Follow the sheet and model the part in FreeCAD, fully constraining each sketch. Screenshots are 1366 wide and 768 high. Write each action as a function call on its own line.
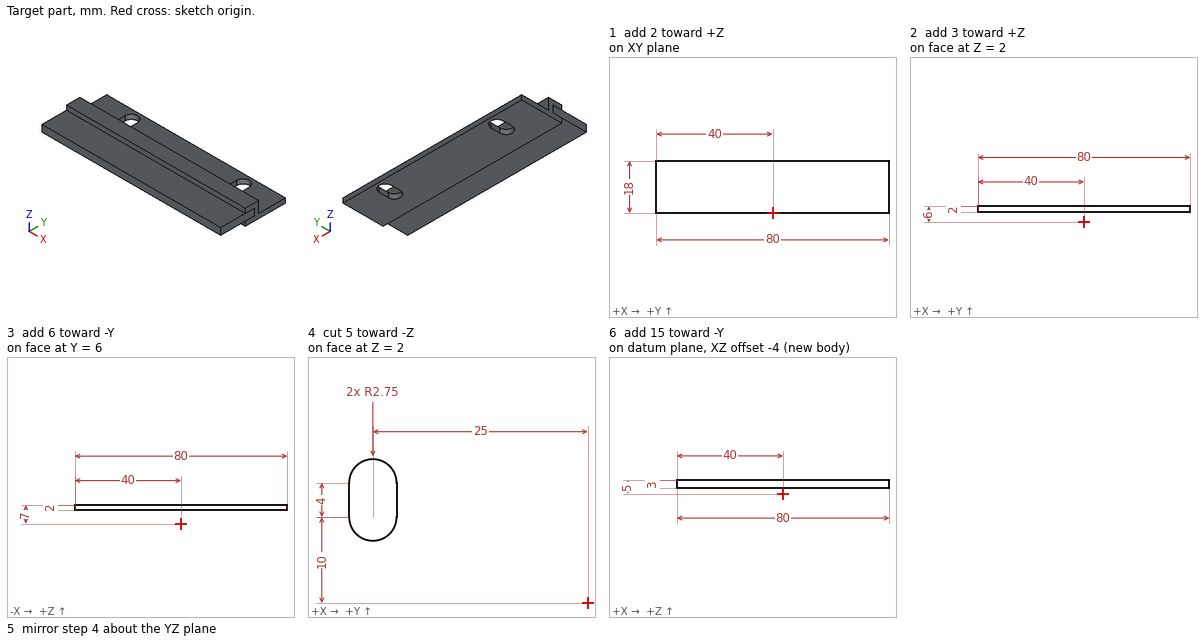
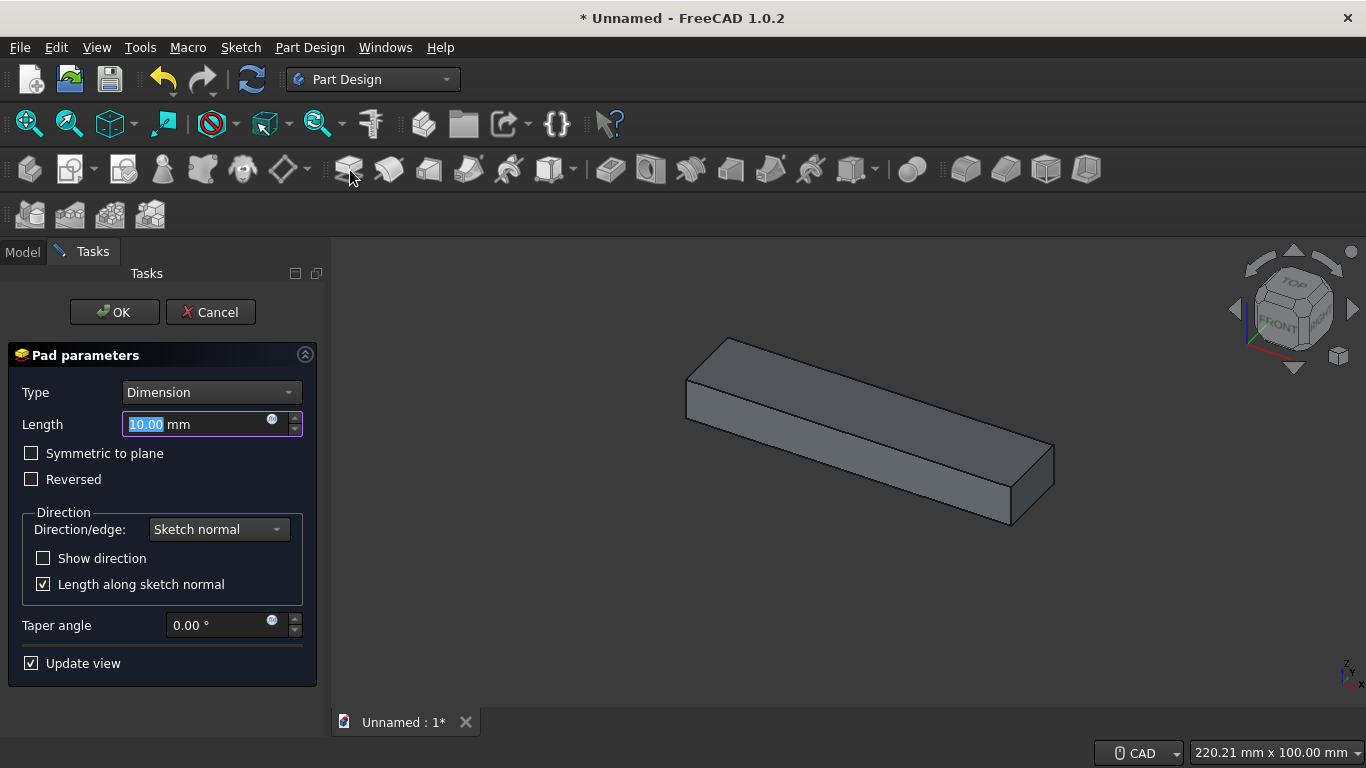
text(2)
key(Tab)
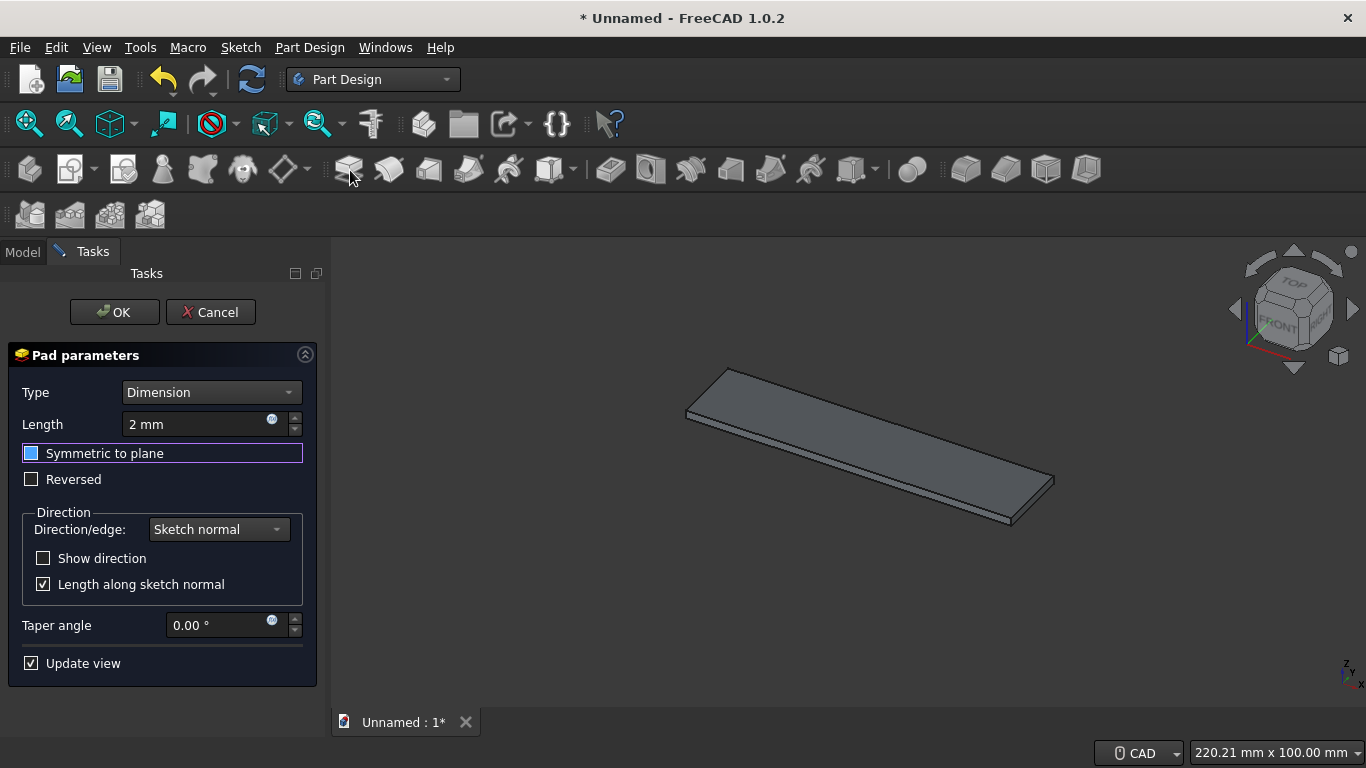
click(115, 312)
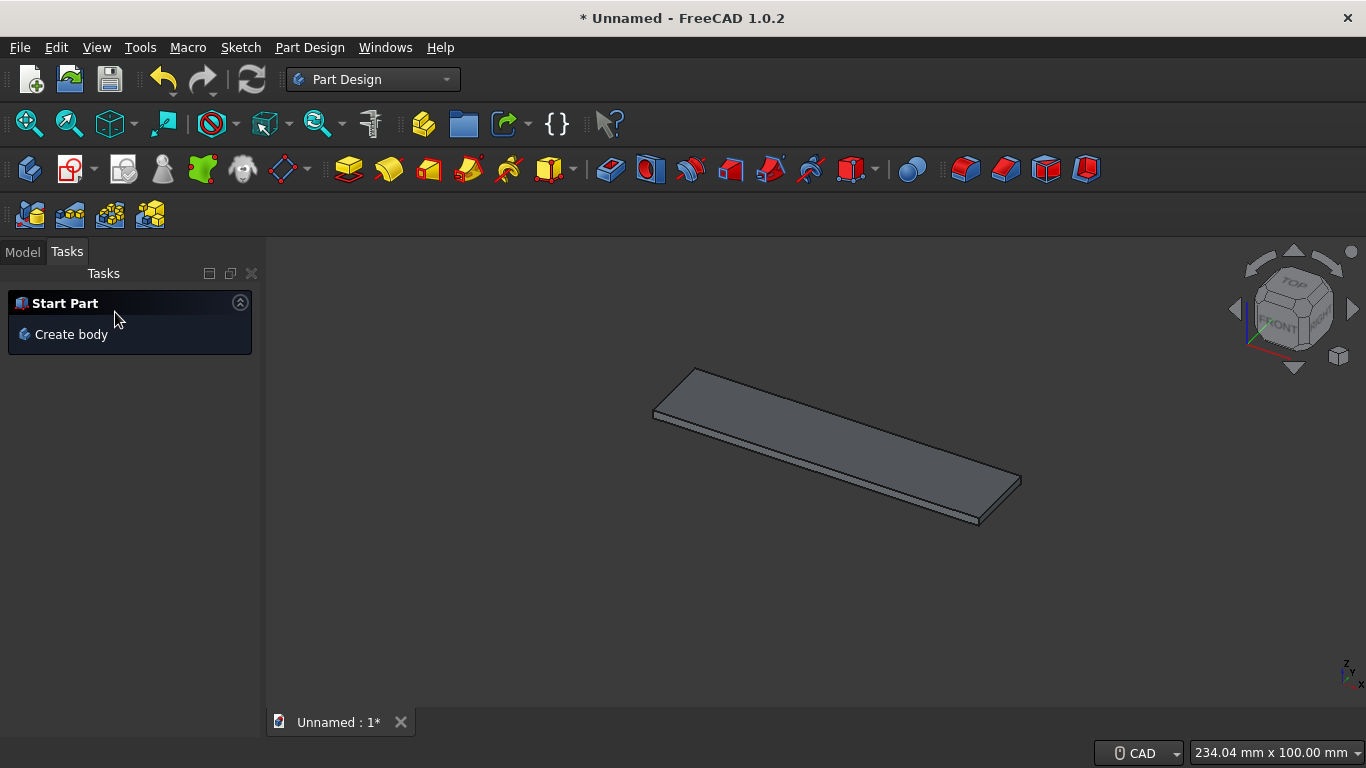
click(30, 124)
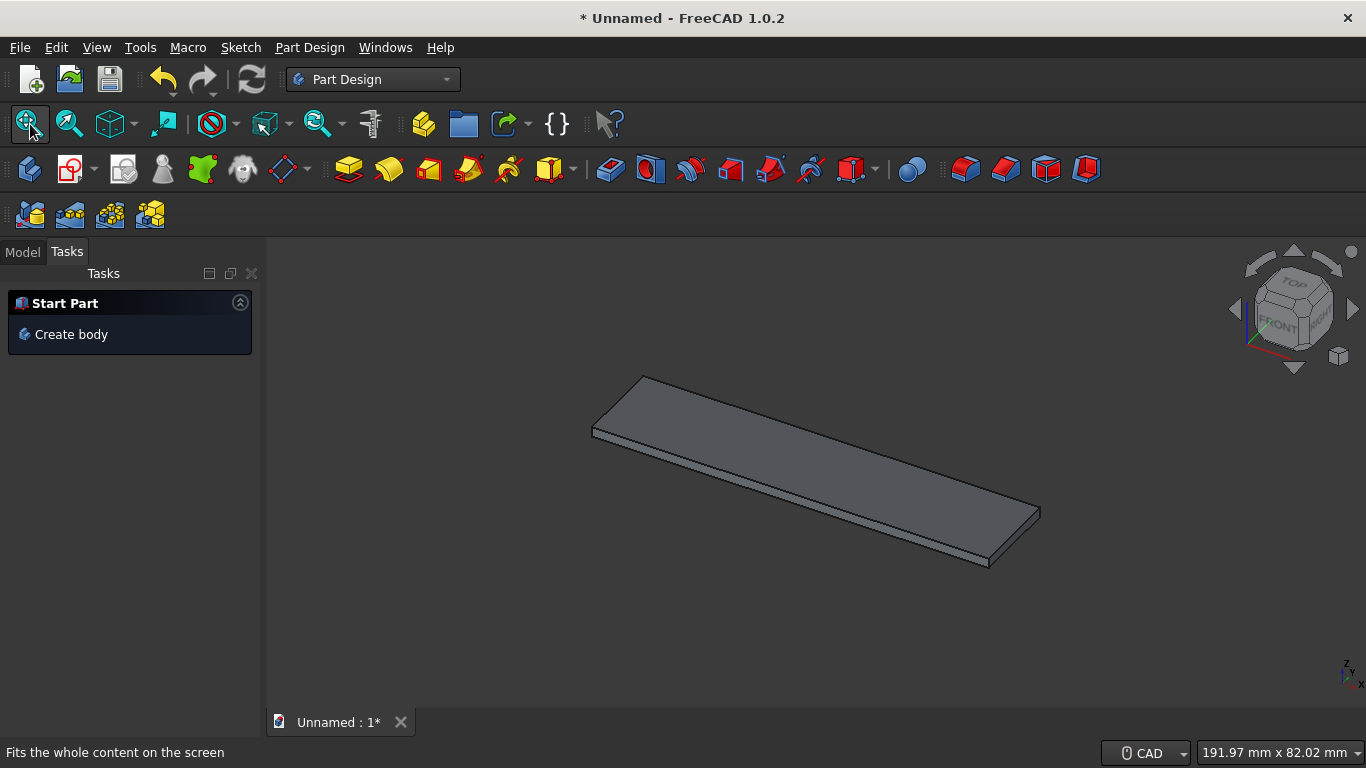
click(929, 504)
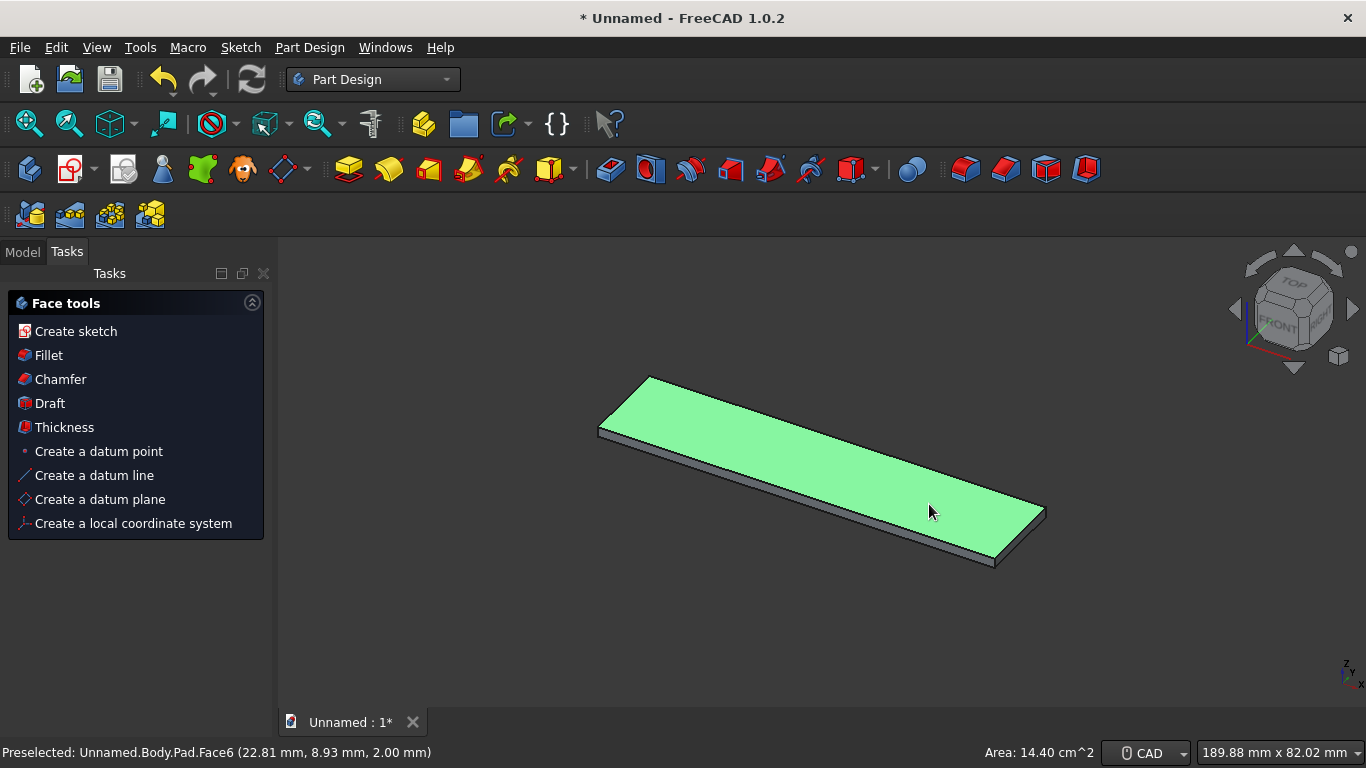
click(70, 170)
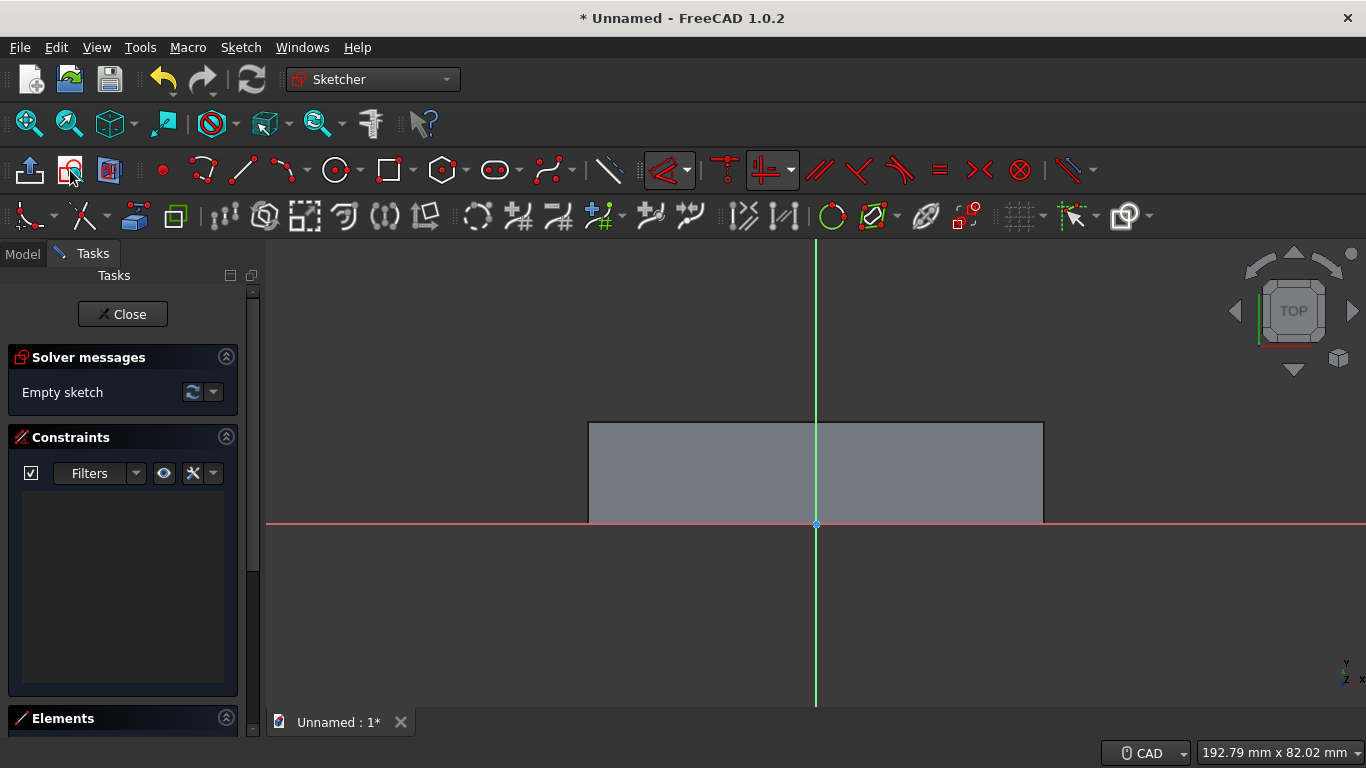
scroll(955, 577, up, 2)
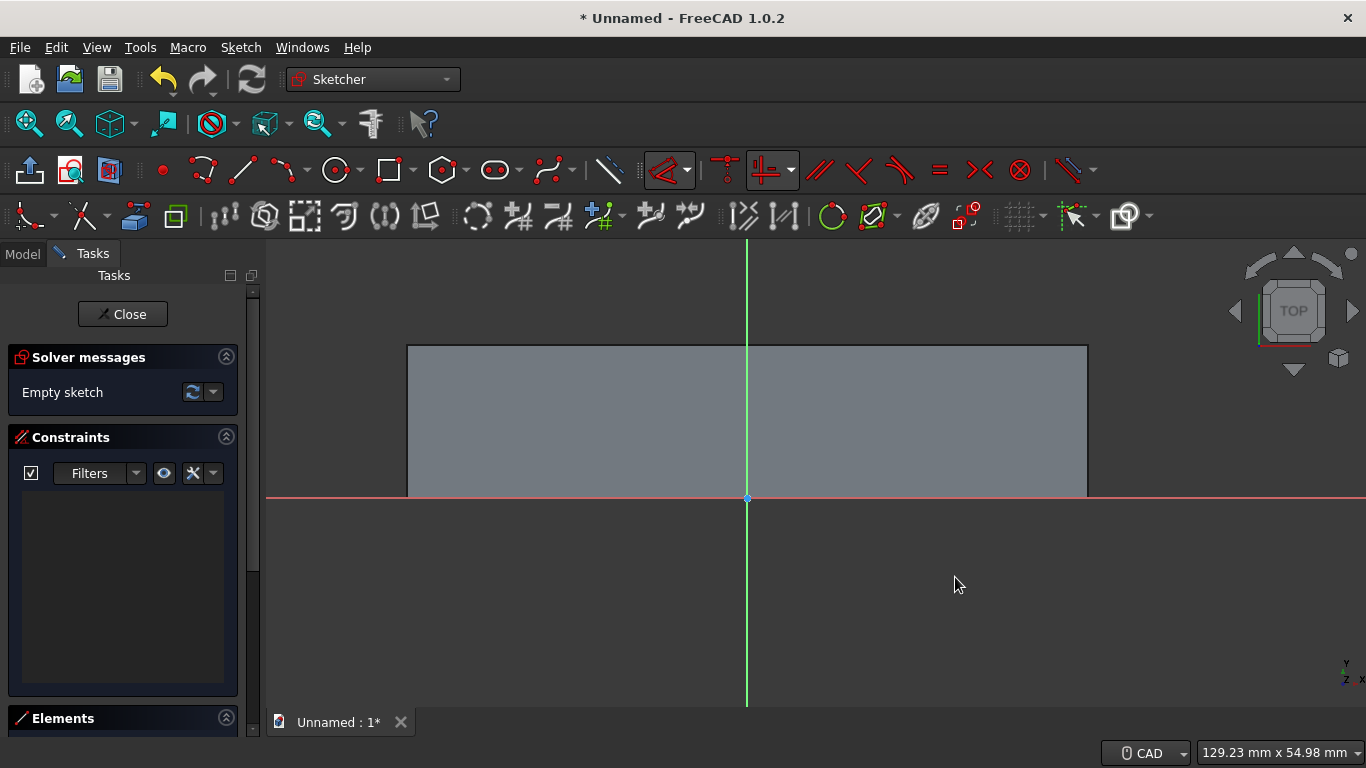
click(390, 170)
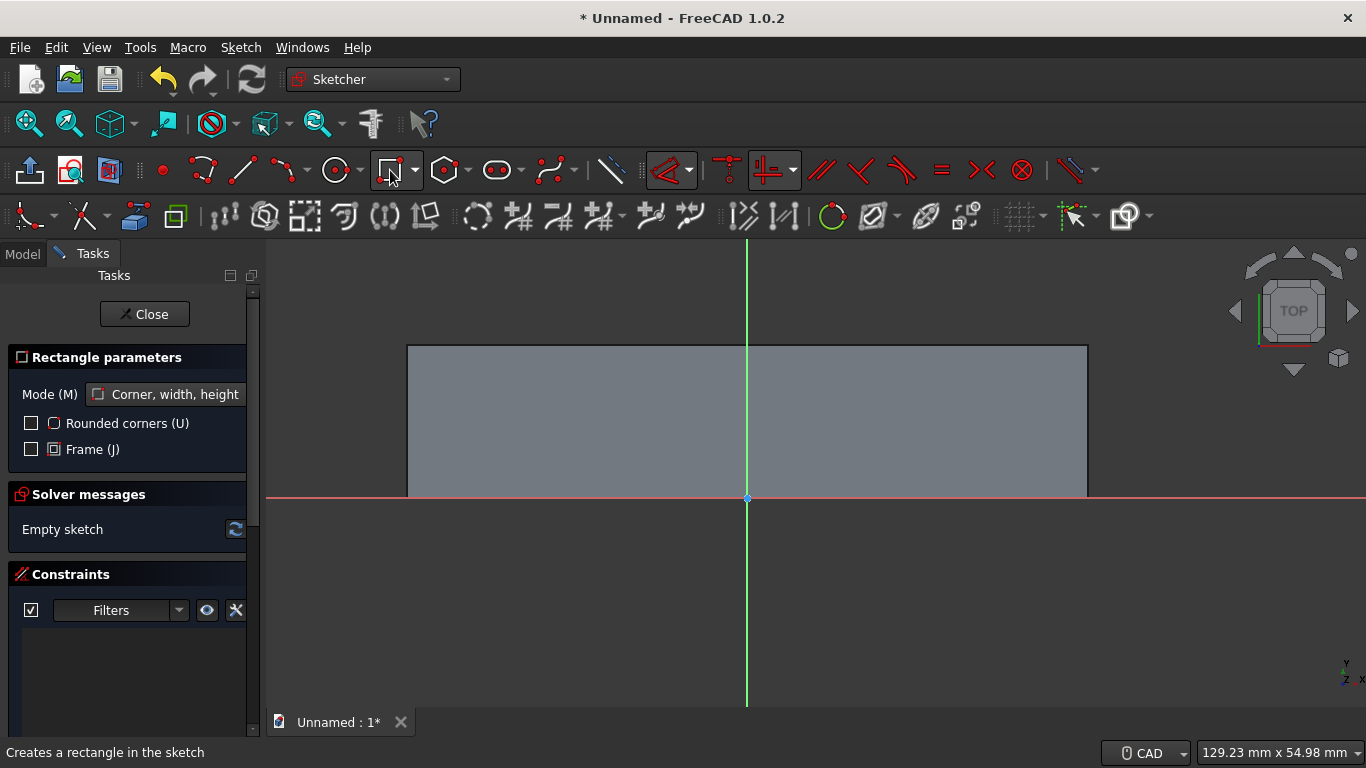
click(407, 447)
click(1088, 464)
key(Escape)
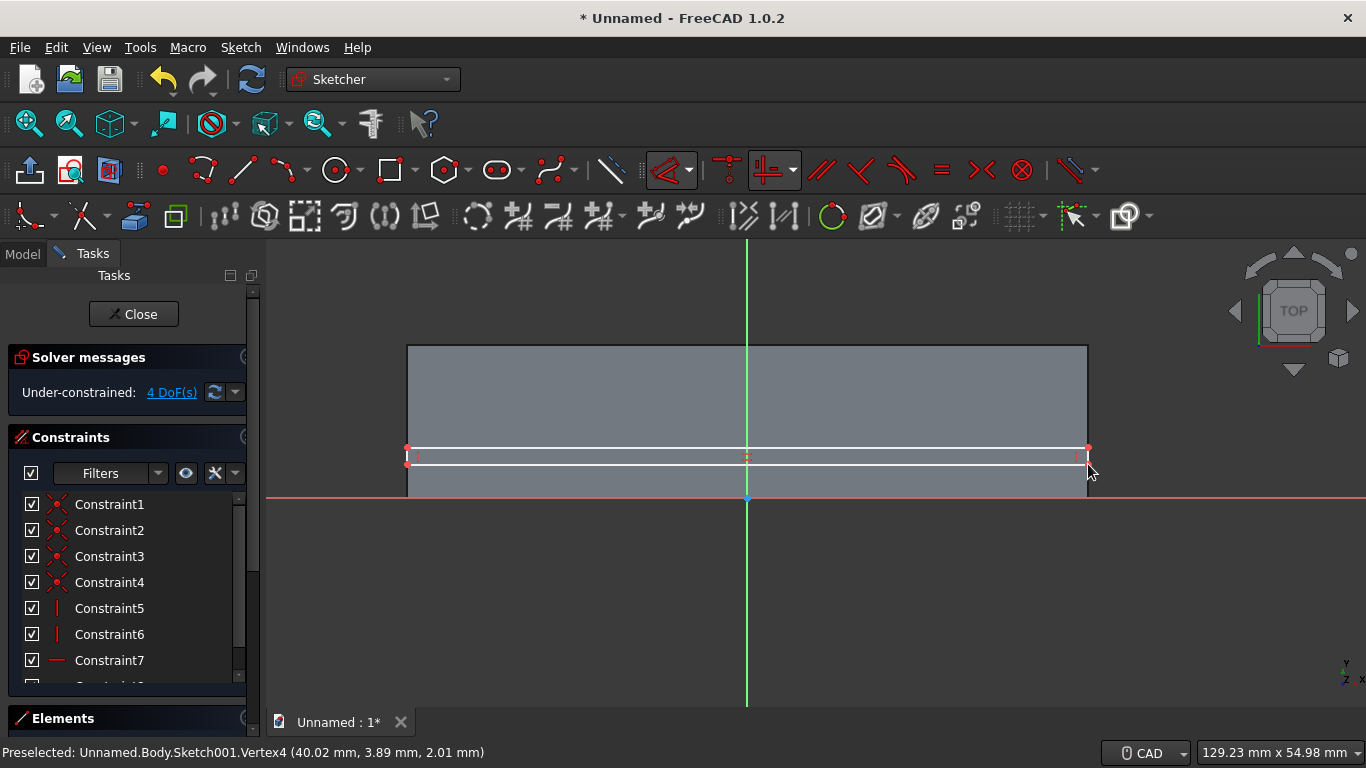
scroll(407, 456, up, 5)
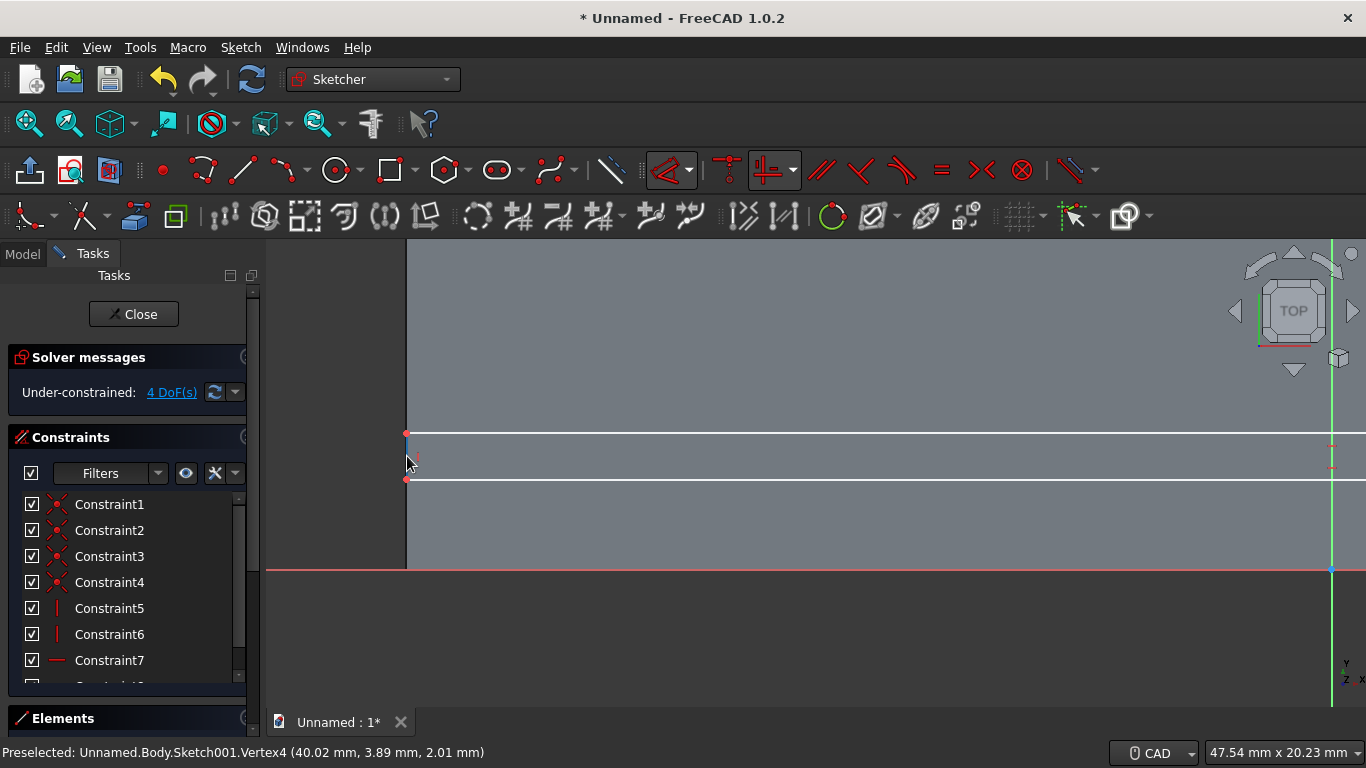
click(407, 457)